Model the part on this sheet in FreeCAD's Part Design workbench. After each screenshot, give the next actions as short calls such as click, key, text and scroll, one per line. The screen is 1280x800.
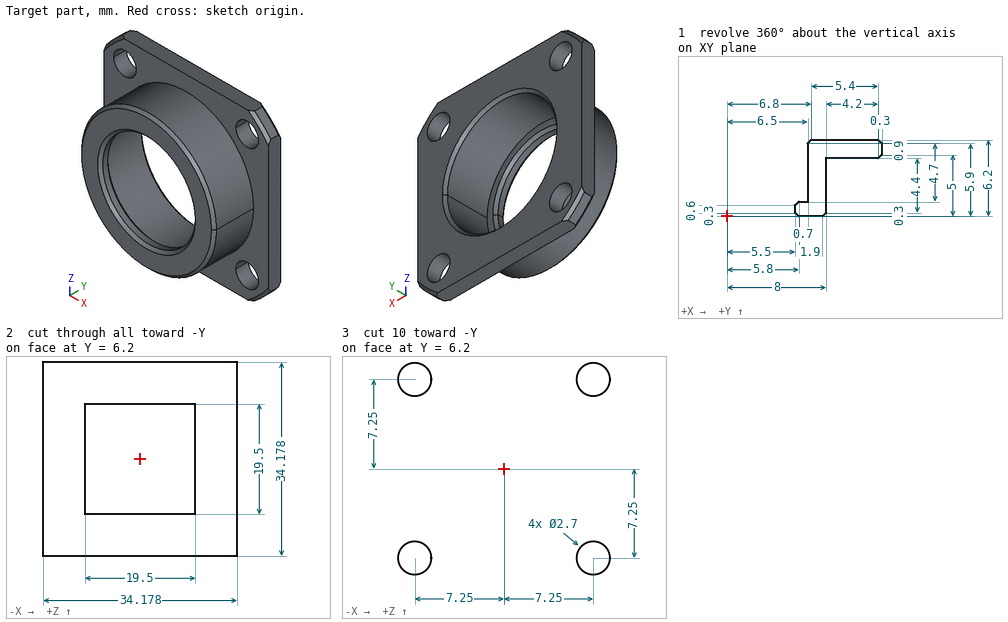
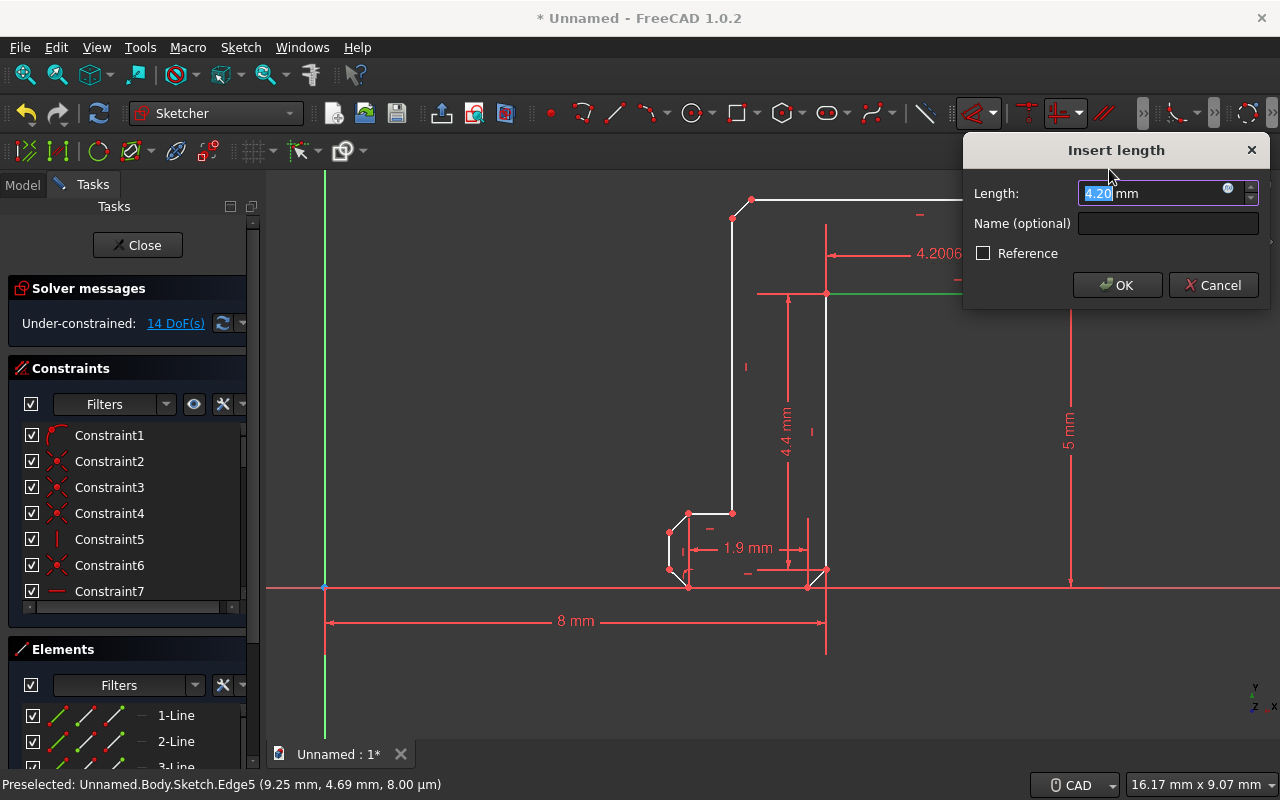
text(4.2)
key(Return)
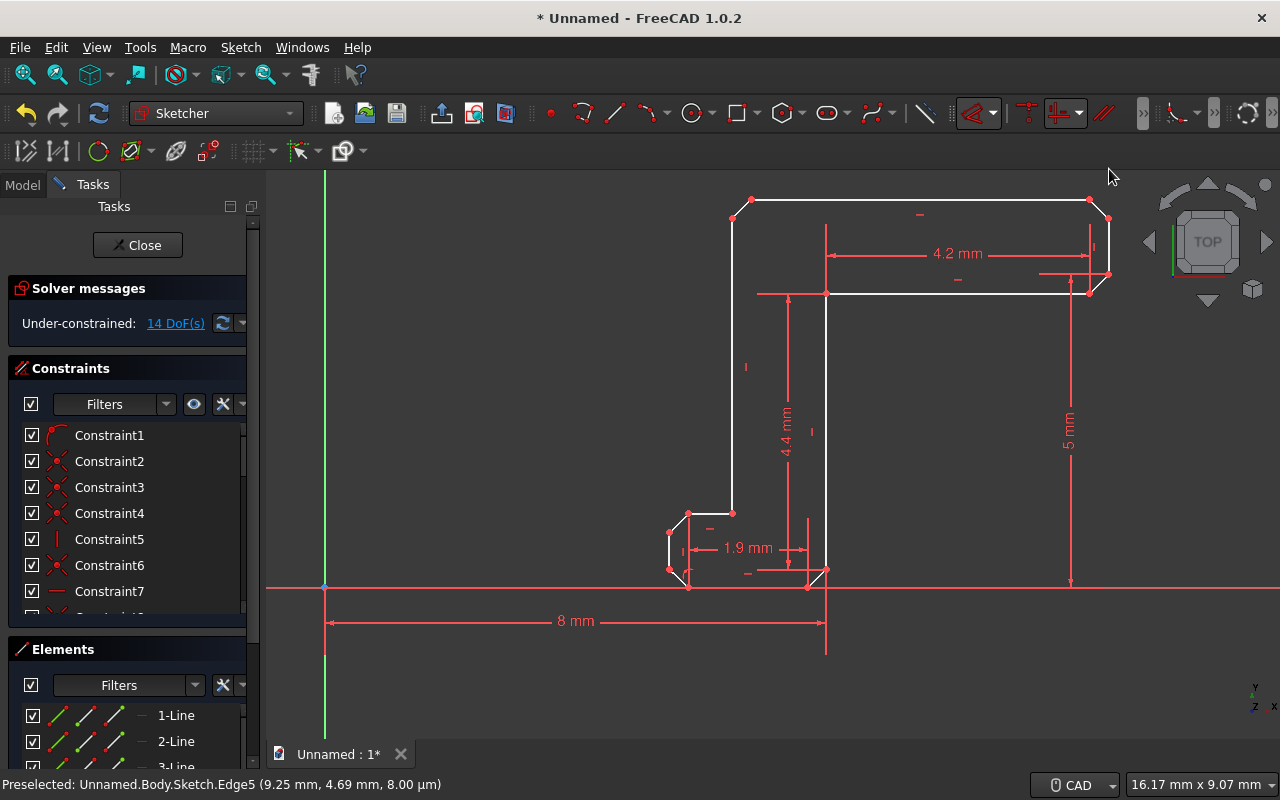
click(1109, 258)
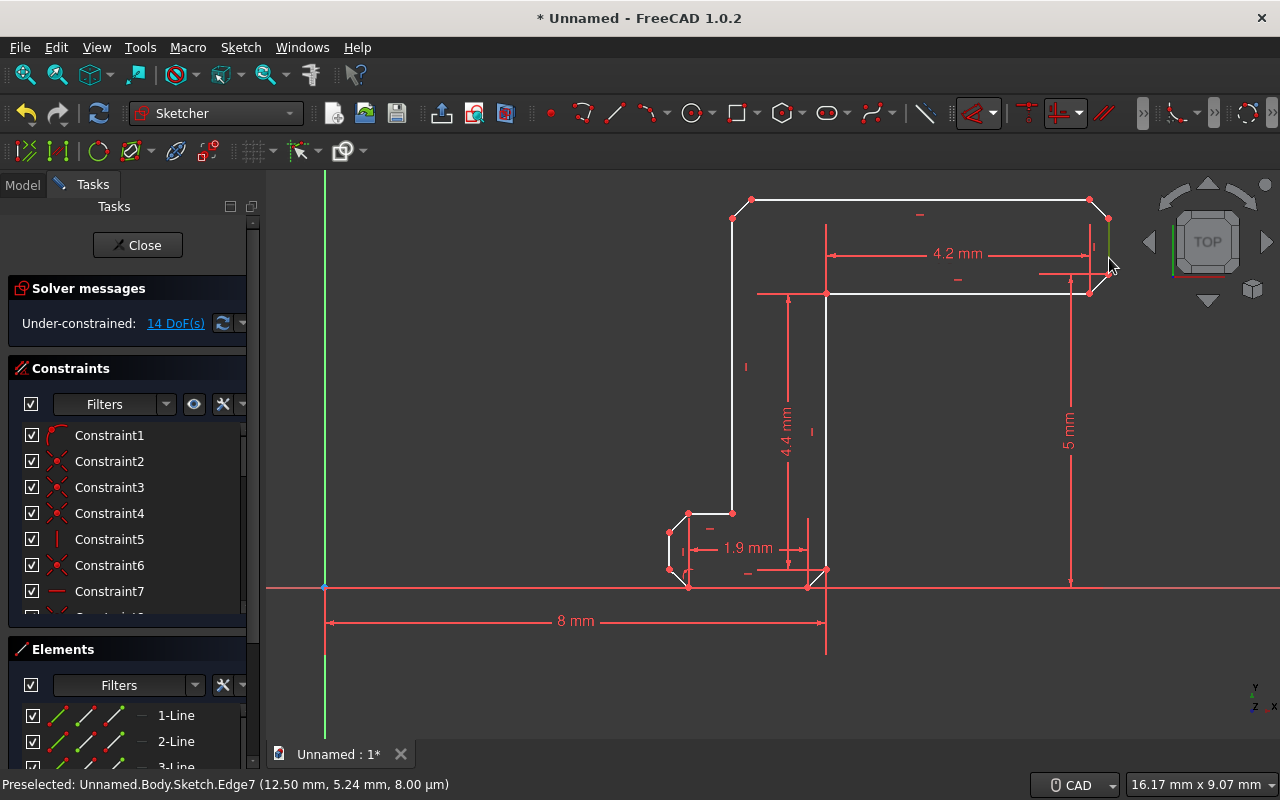
click(996, 114)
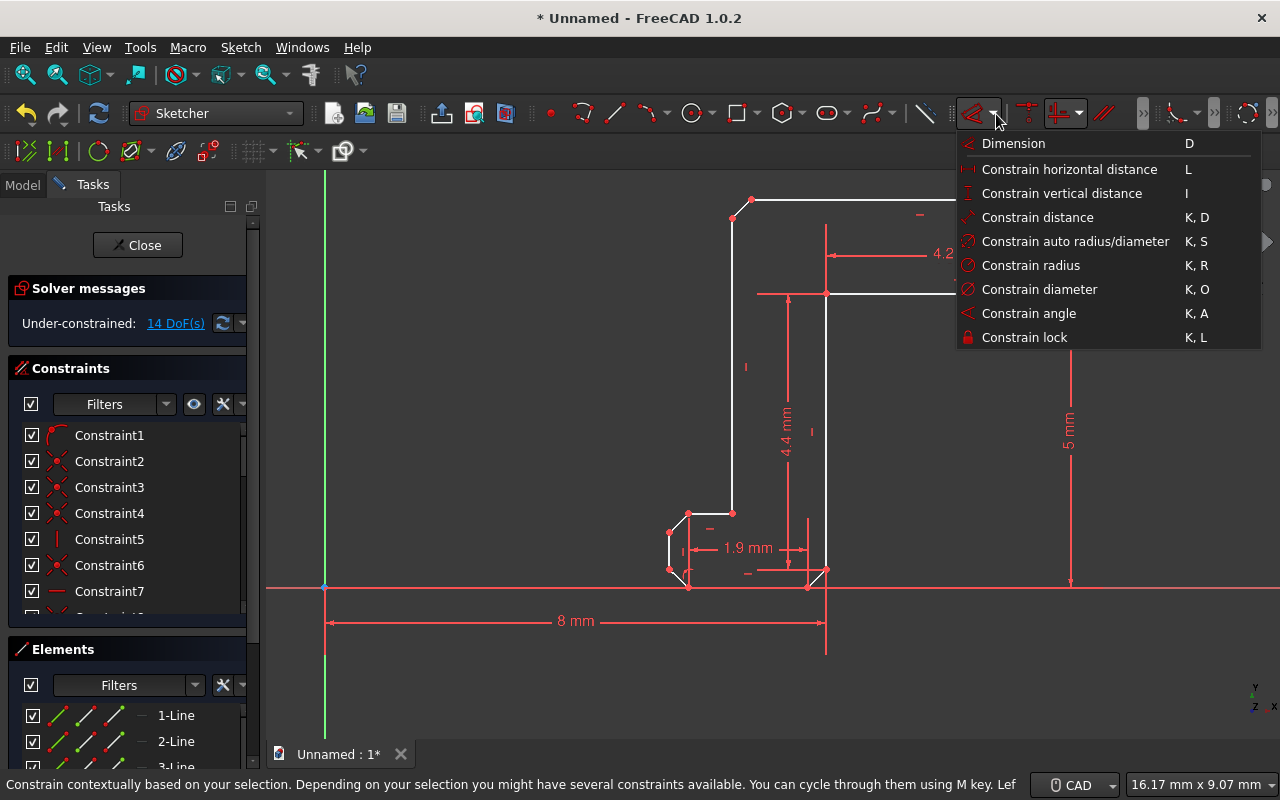
click(1109, 193)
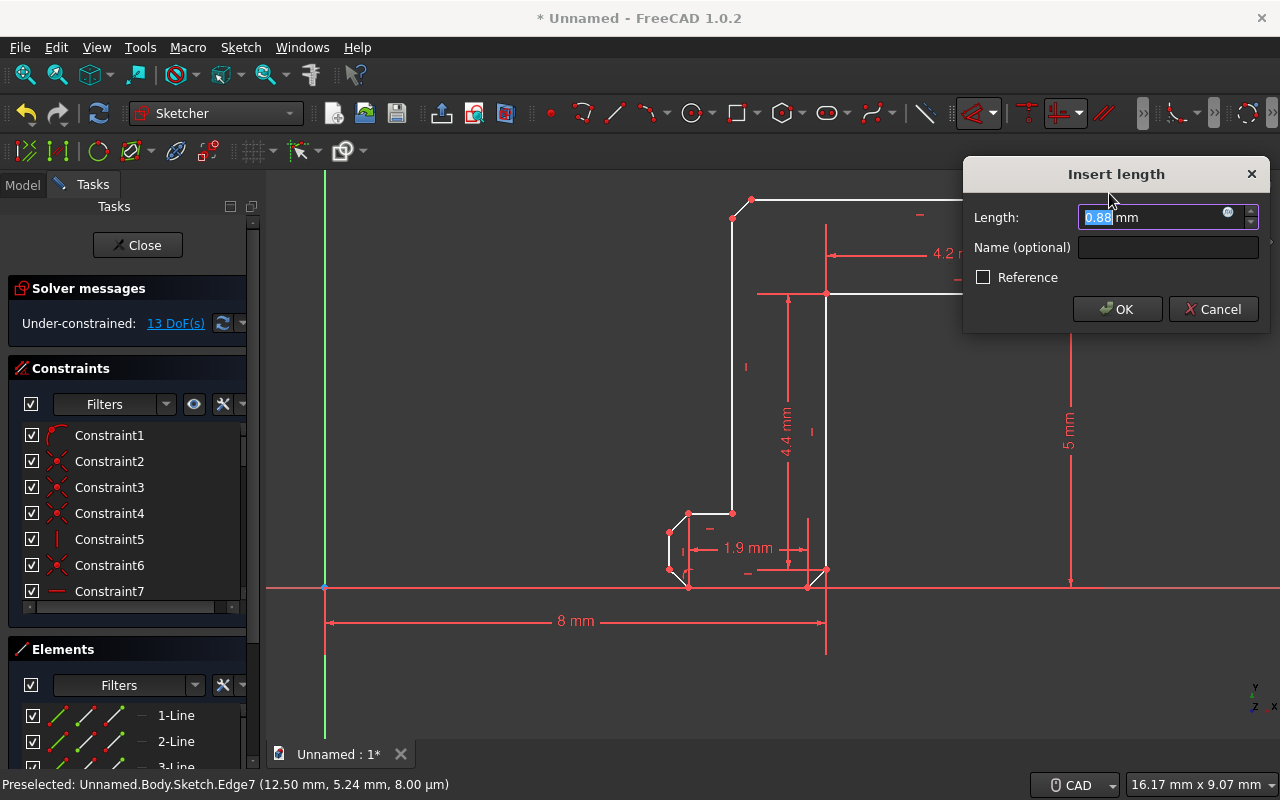
text(0.9)
key(Return)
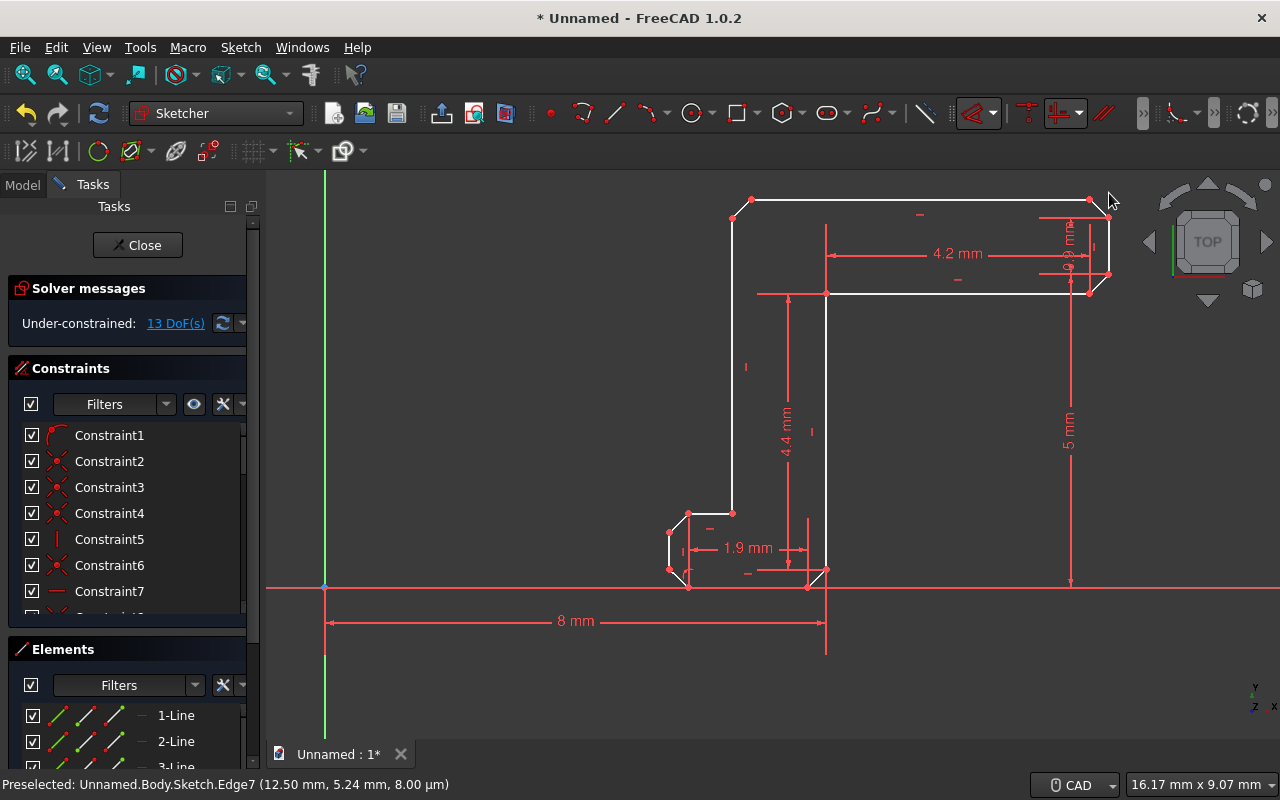
click(988, 200)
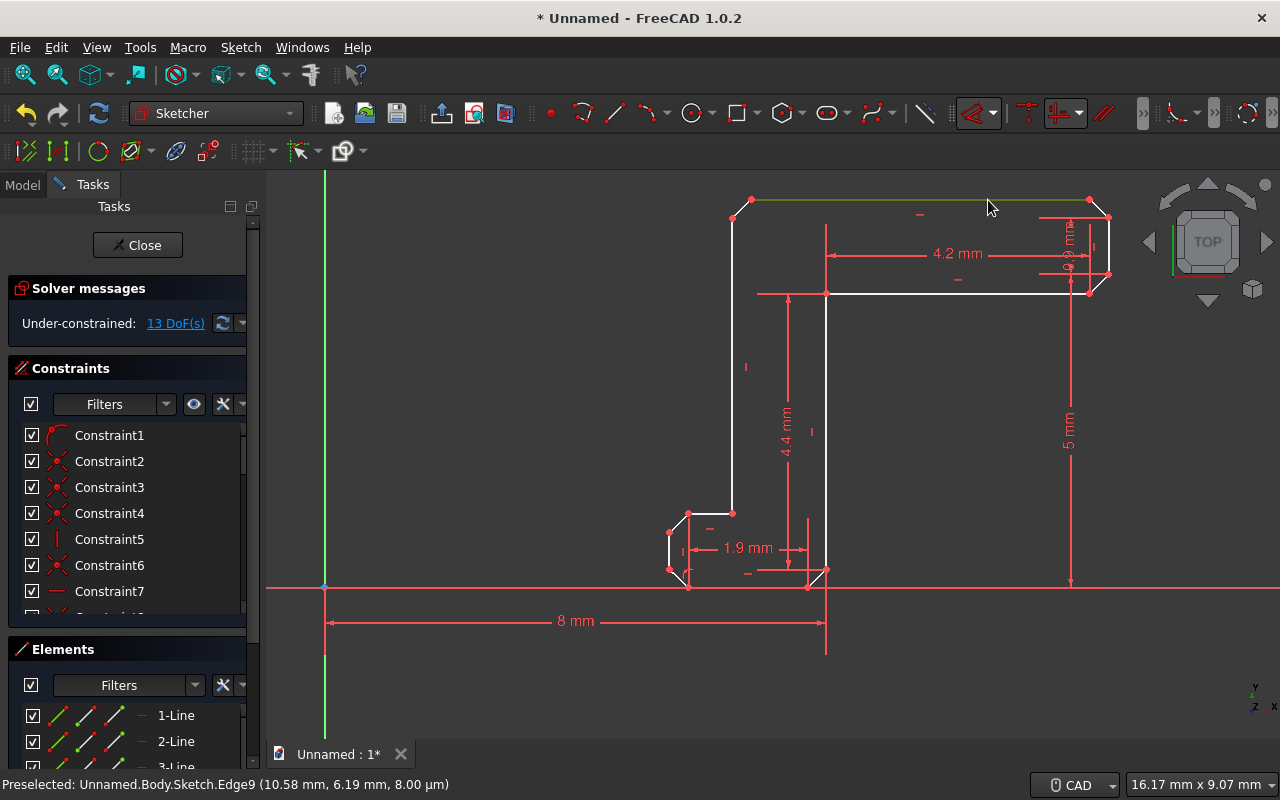
key(l)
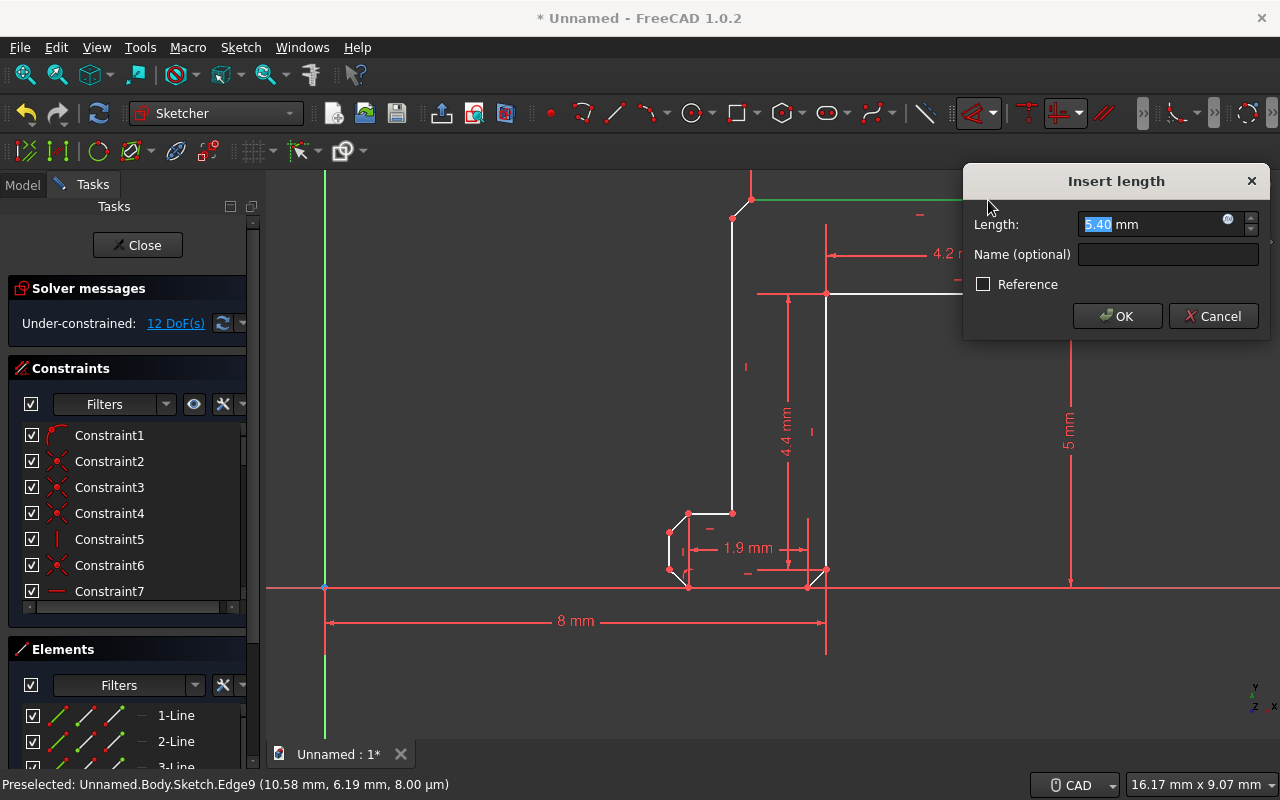
text(5.4)
key(Return)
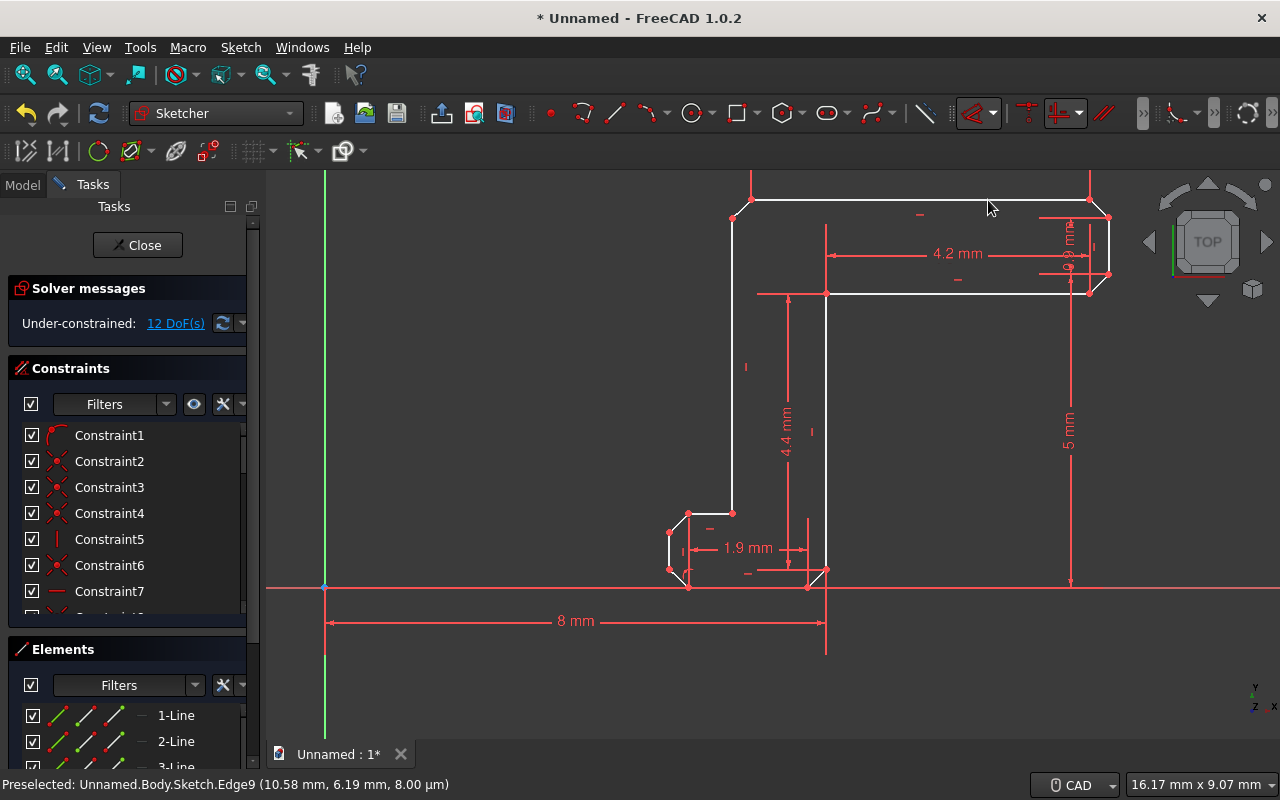
click(732, 307)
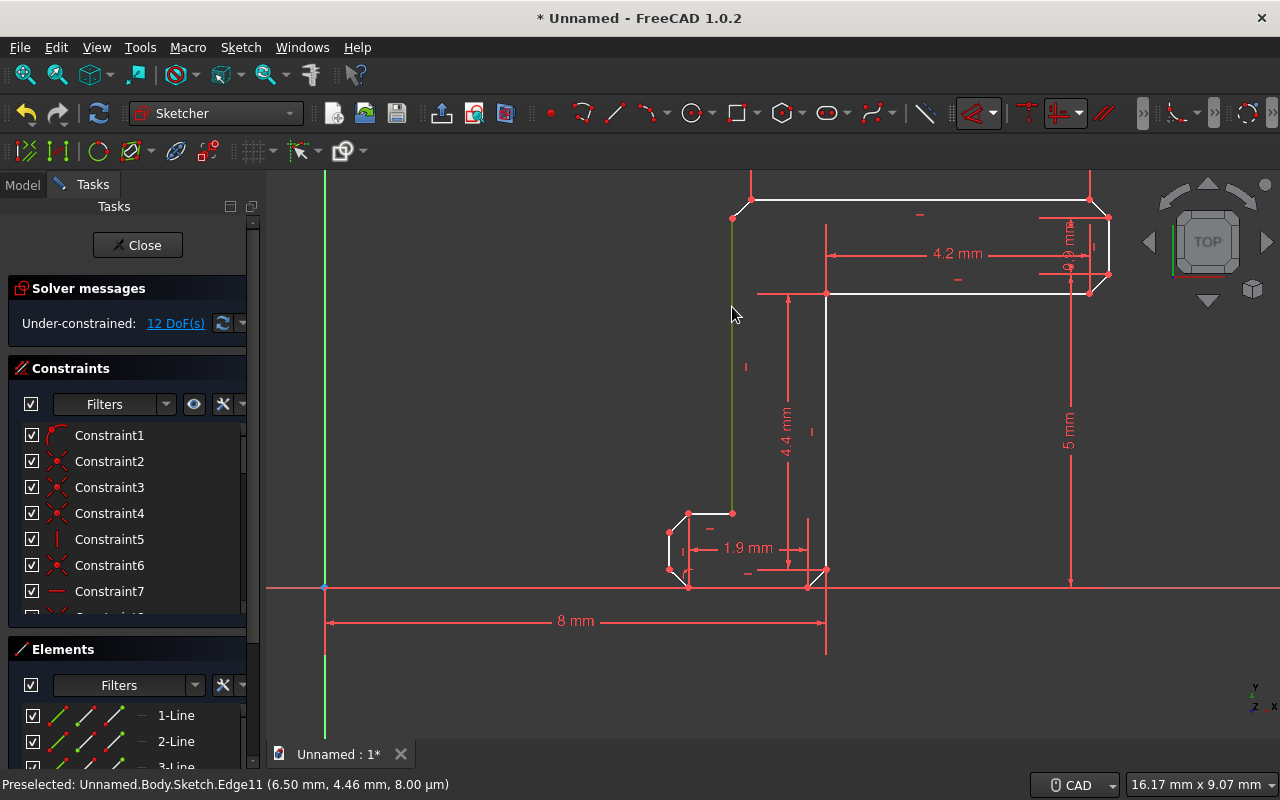
click(996, 114)